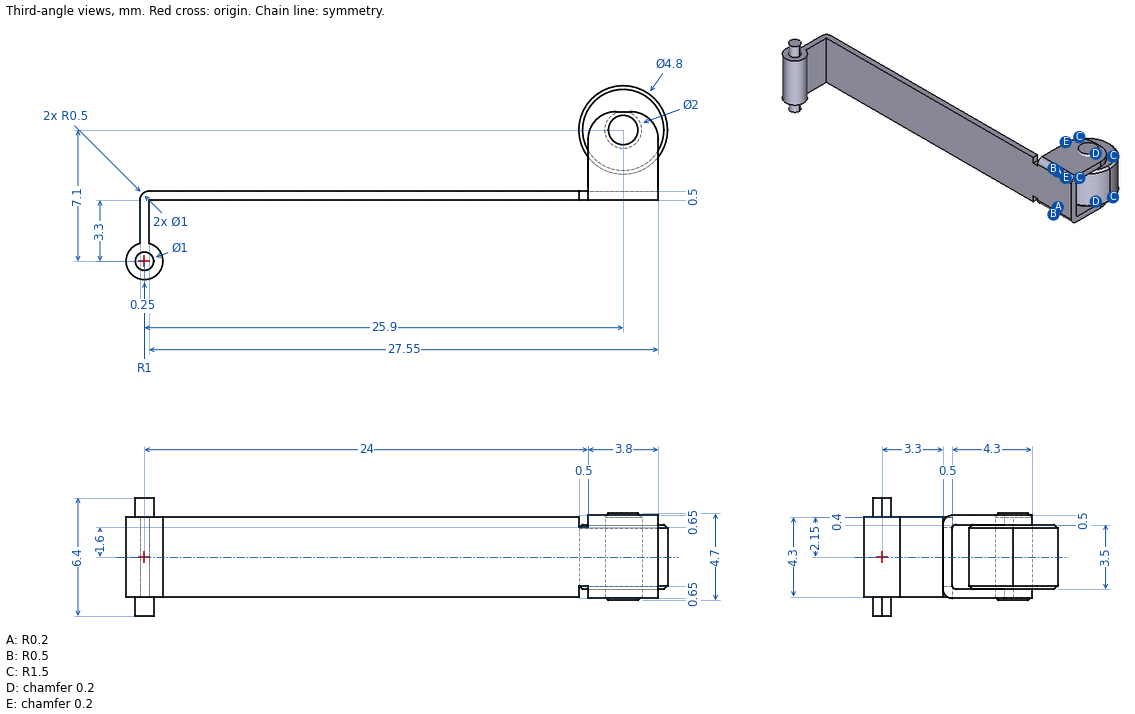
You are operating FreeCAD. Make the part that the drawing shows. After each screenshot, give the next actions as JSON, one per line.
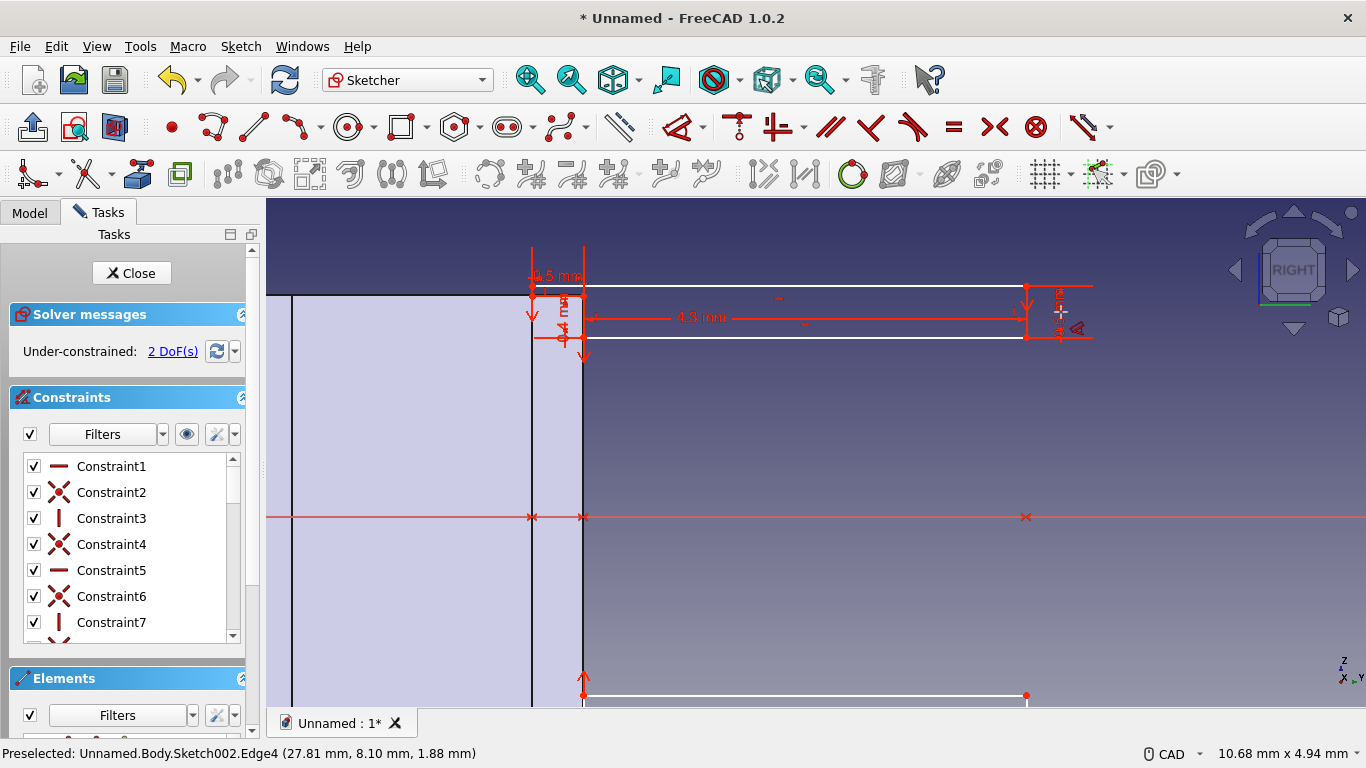
{"action": "left_click", "coordinate": [532, 296]}
{"action": "left_click", "coordinate": [413, 262]}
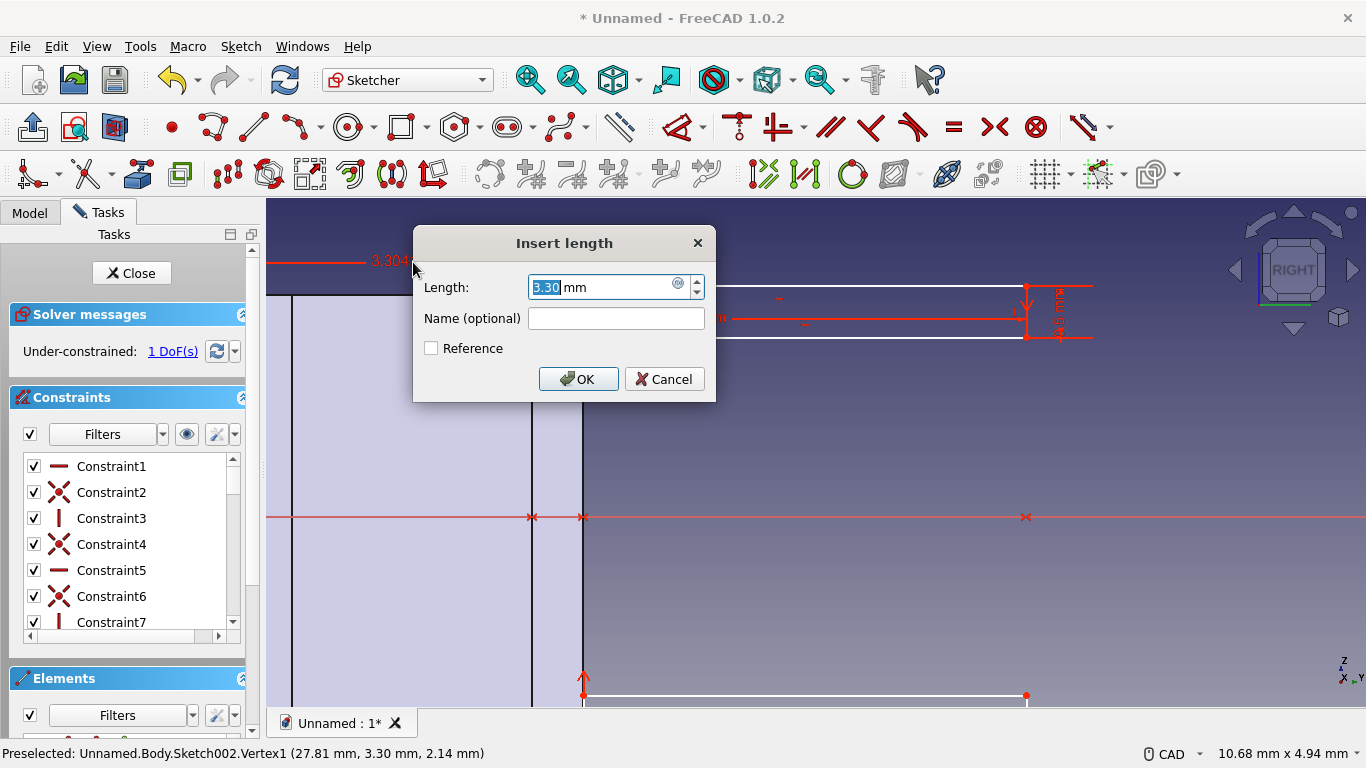
{"action": "type", "text": "3.3"}
{"action": "key", "text": "Return"}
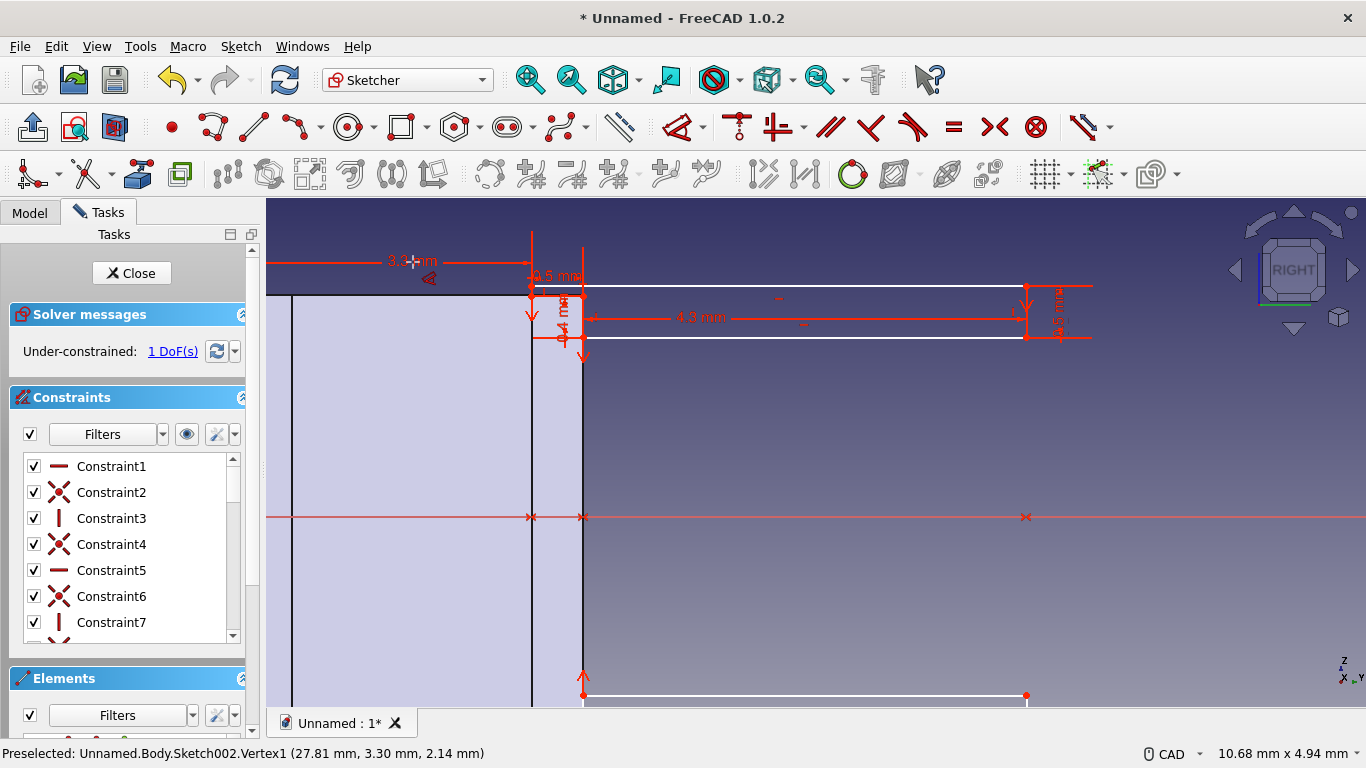
{"action": "left_click", "coordinate": [532, 296]}
{"action": "left_click", "coordinate": [566, 406]}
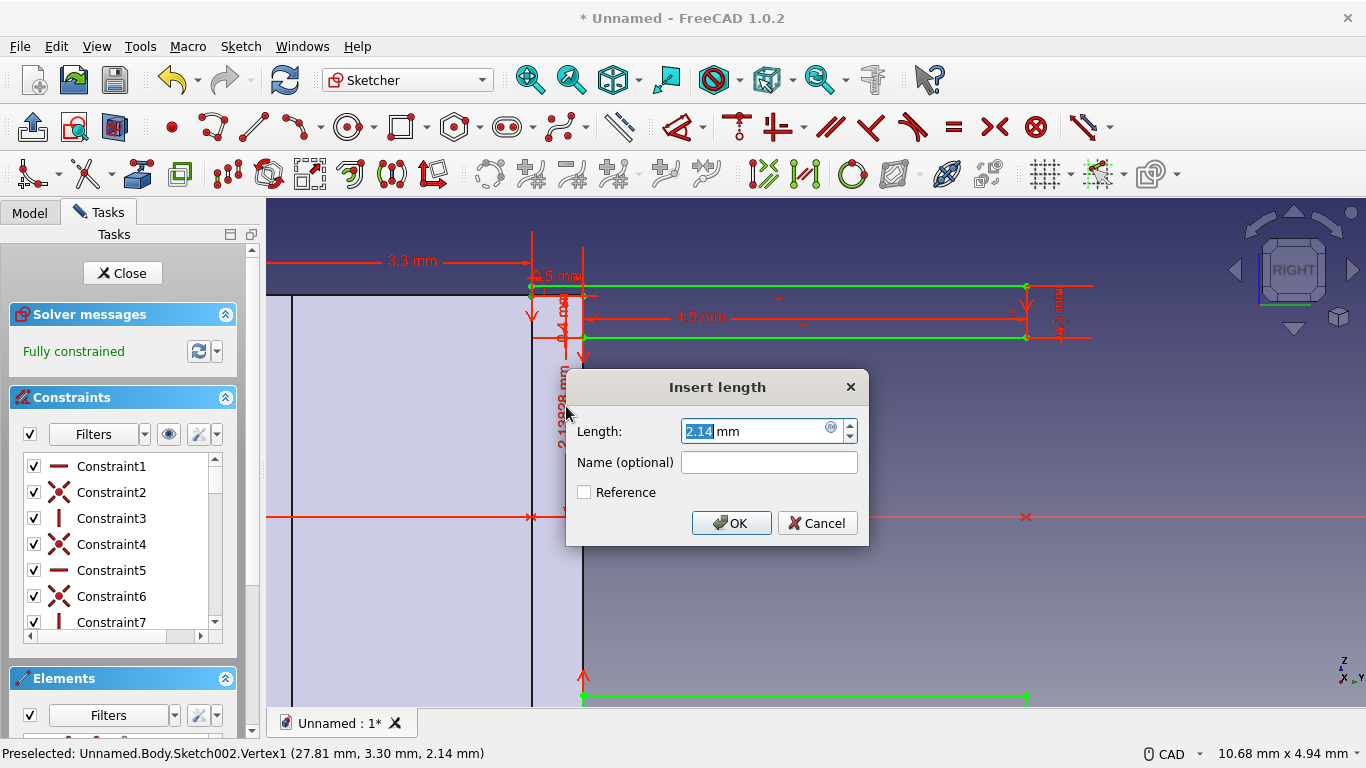
{"action": "type", "text": "2.15"}
{"action": "key", "text": "Return"}
{"action": "key", "text": "Escape"}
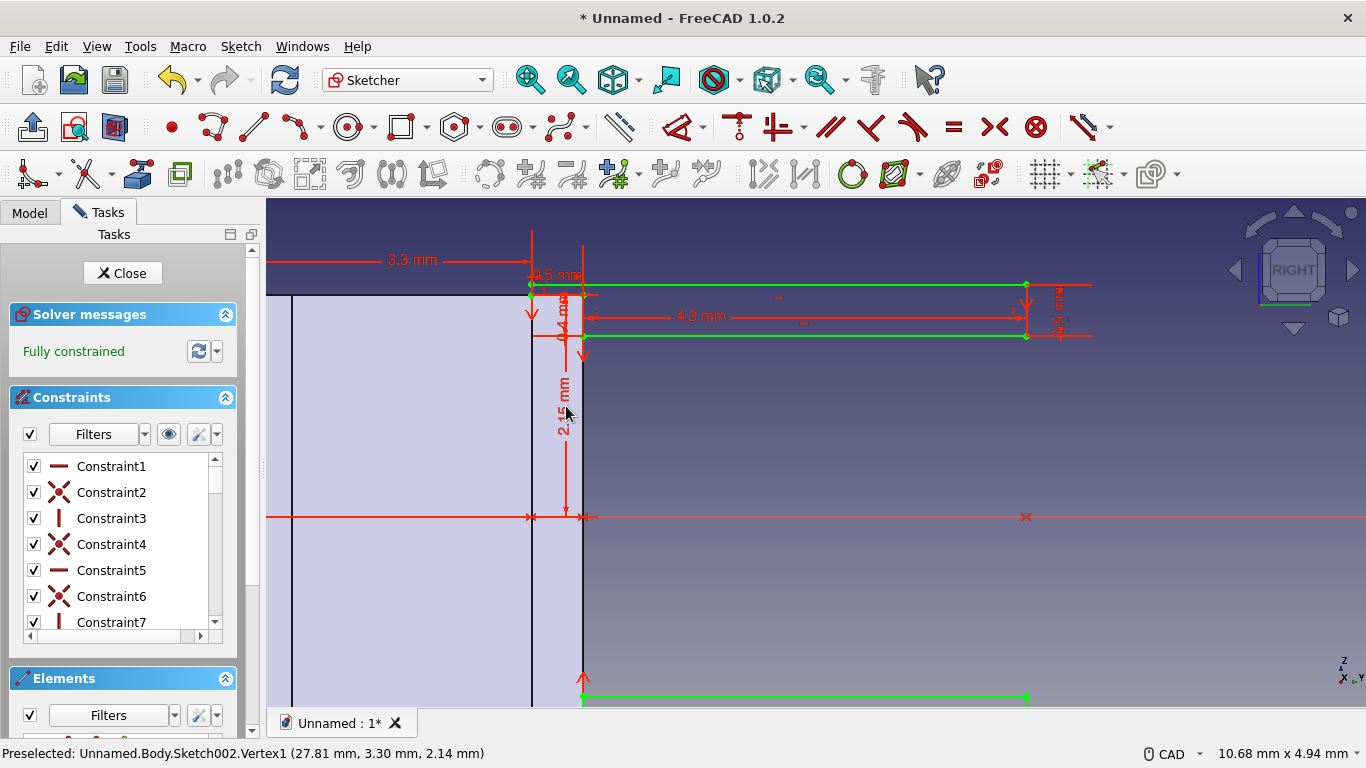
{"action": "left_click", "coordinate": [123, 273]}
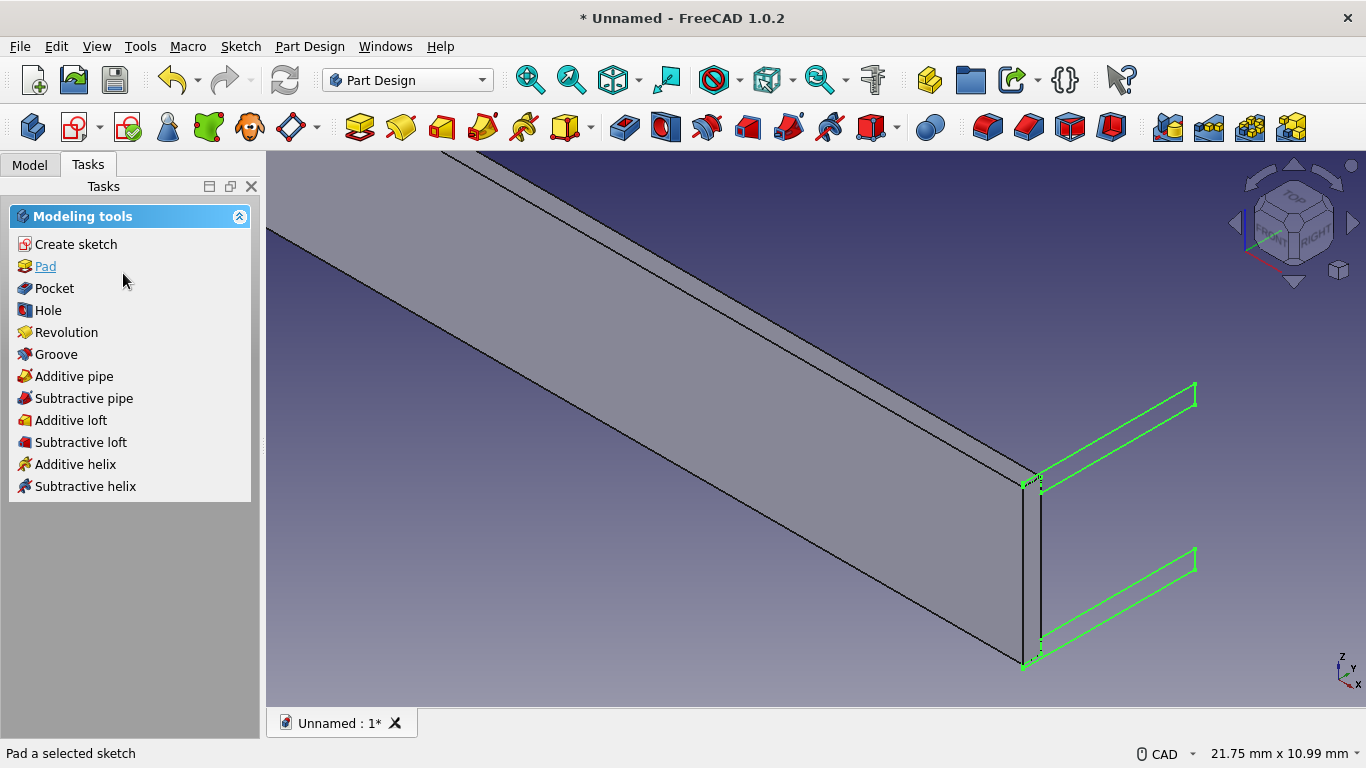
{"action": "left_click", "coordinate": [360, 128]}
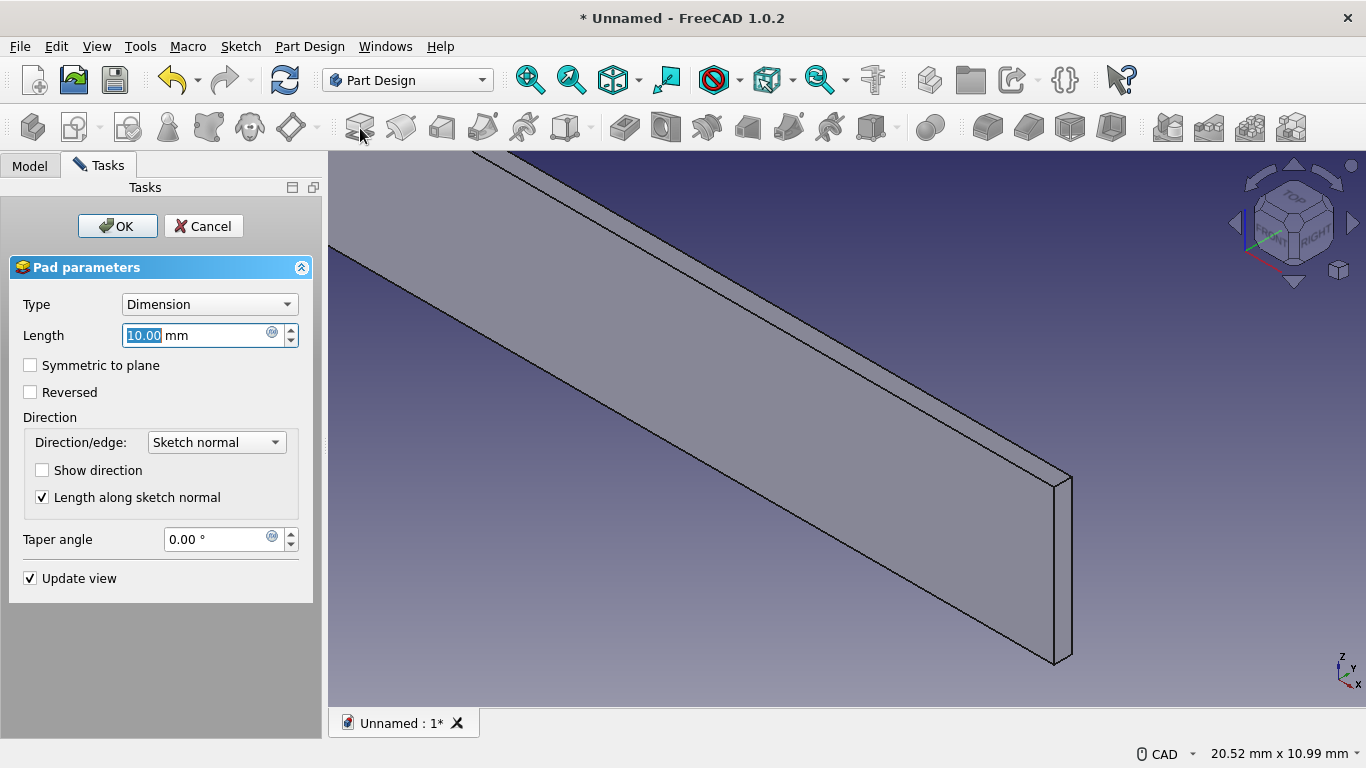
{"action": "type", "text": "3.8"}
{"action": "key", "text": "Tab"}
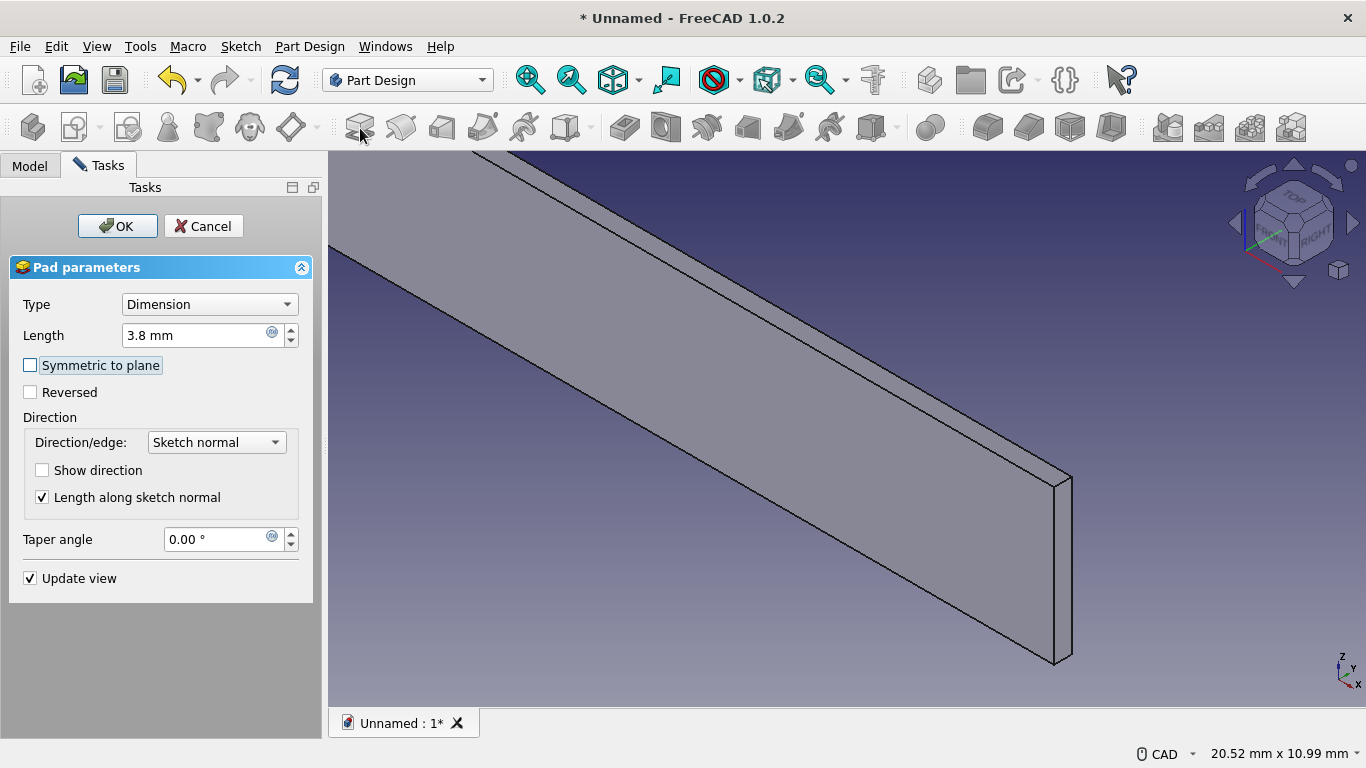
{"action": "left_click", "coordinate": [31, 392]}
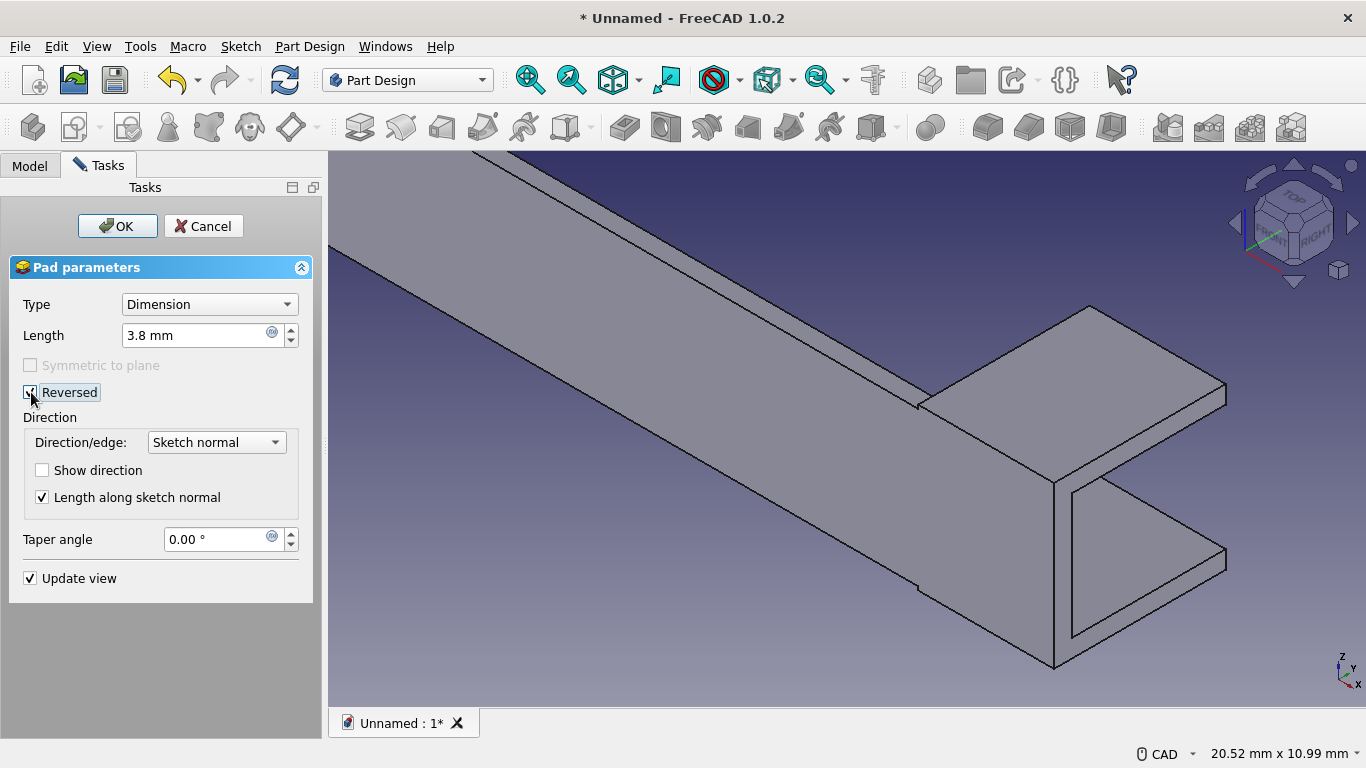
{"action": "left_click", "coordinate": [118, 226]}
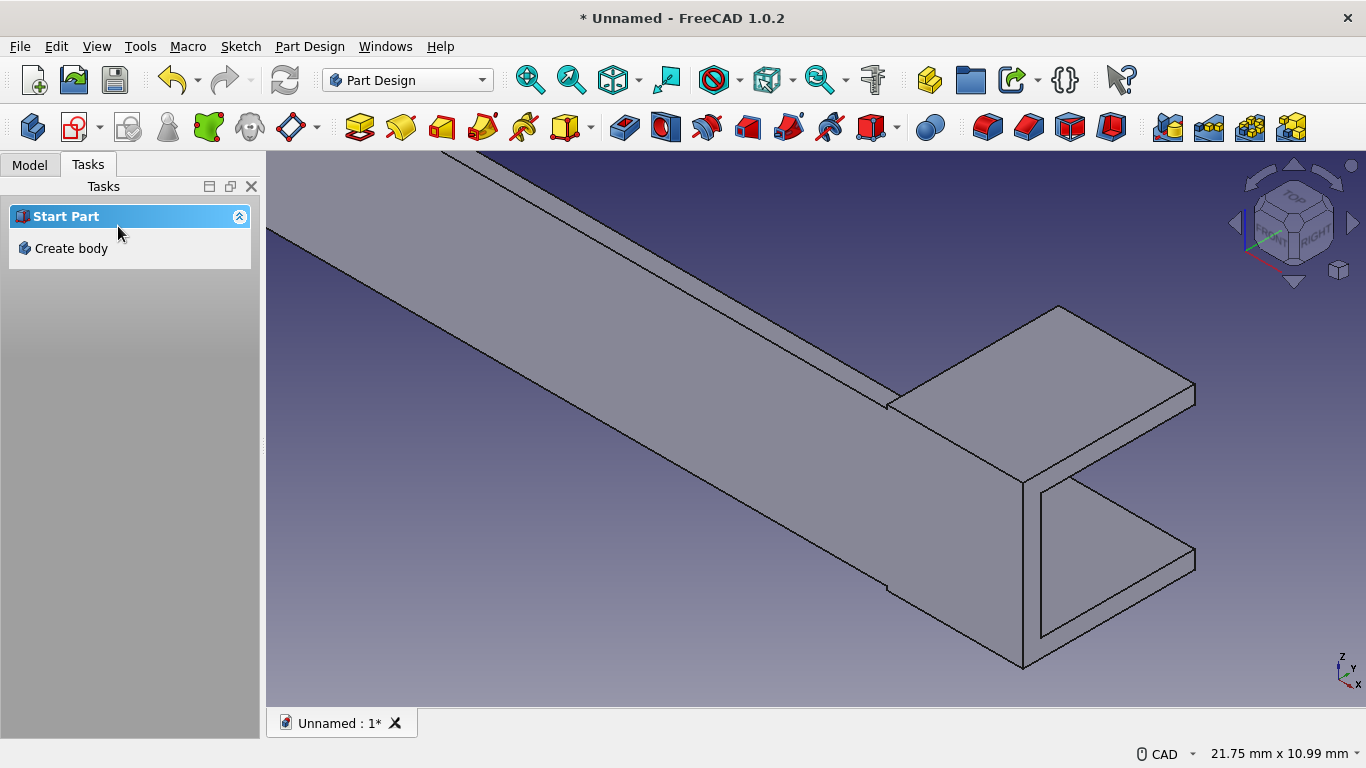
{"action": "left_click", "coordinate": [531, 80]}